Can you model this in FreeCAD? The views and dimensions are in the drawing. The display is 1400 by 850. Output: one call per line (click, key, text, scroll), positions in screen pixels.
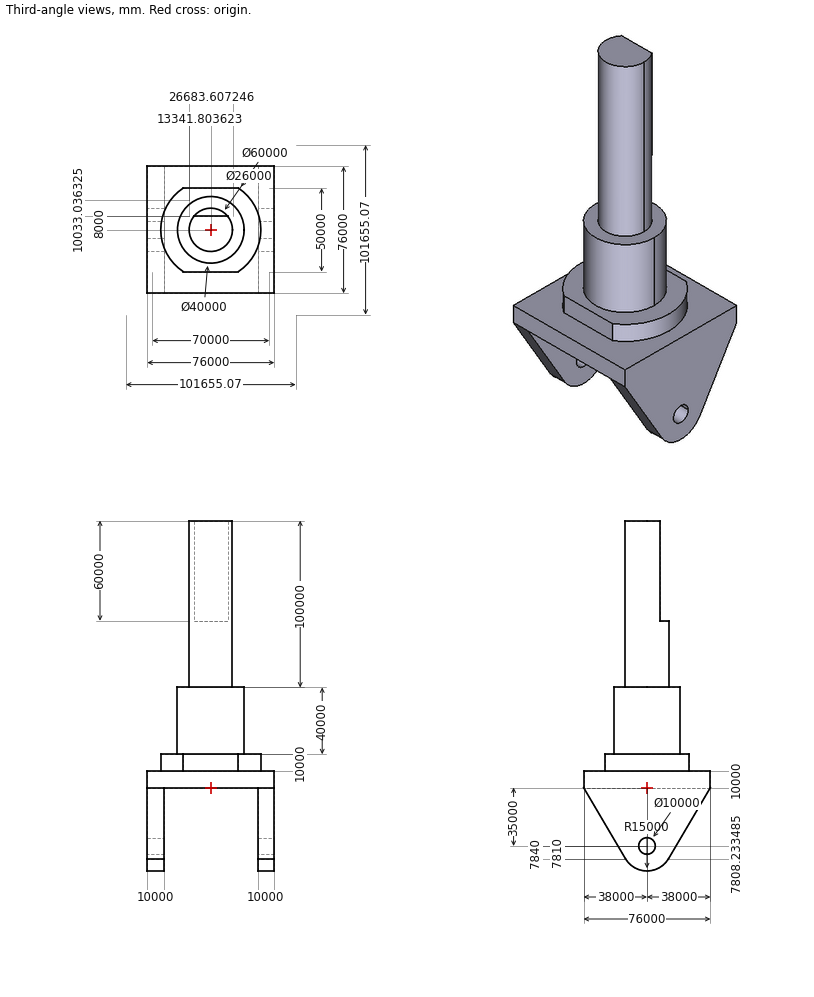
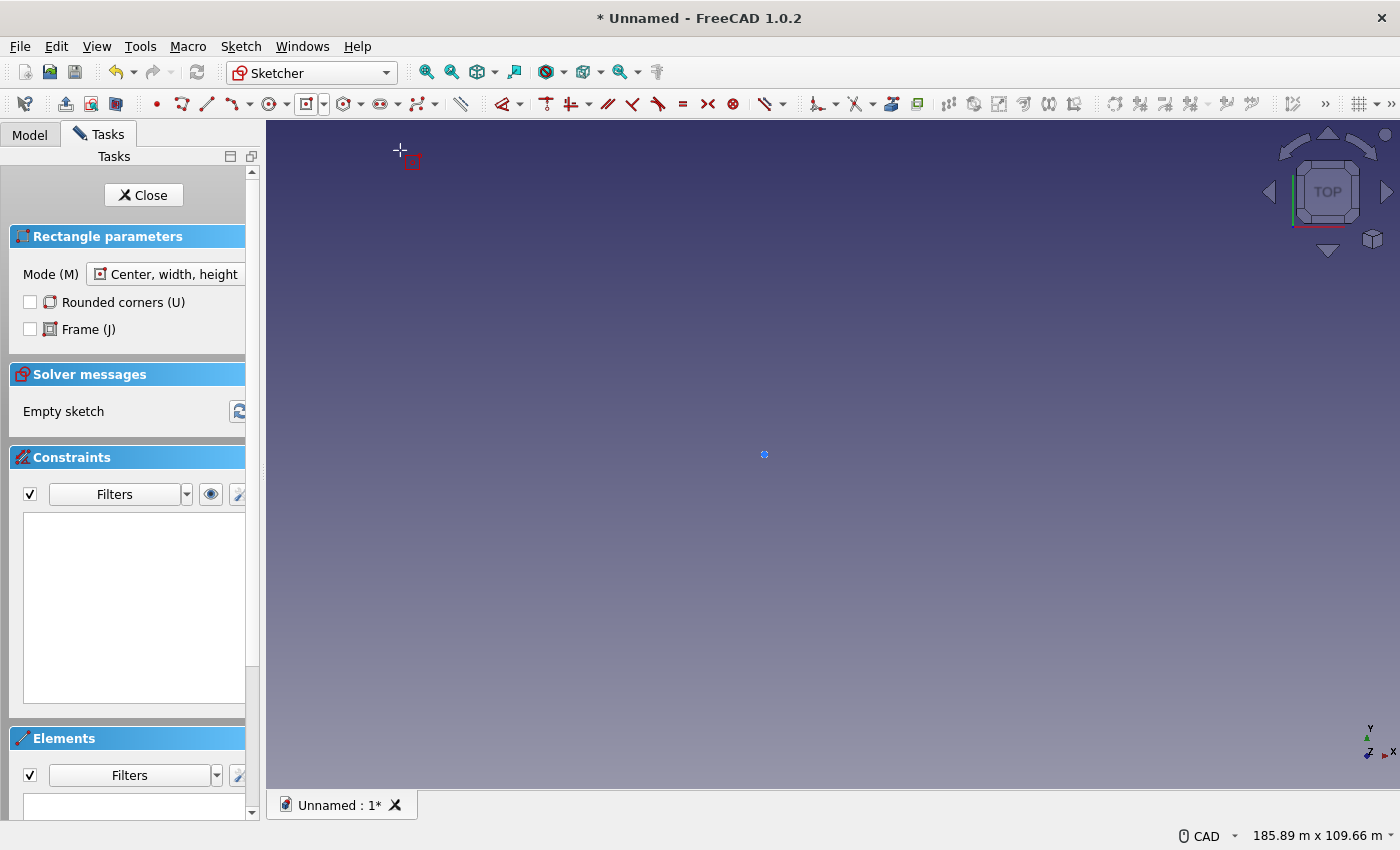
click(765, 454)
click(996, 223)
key(Escape)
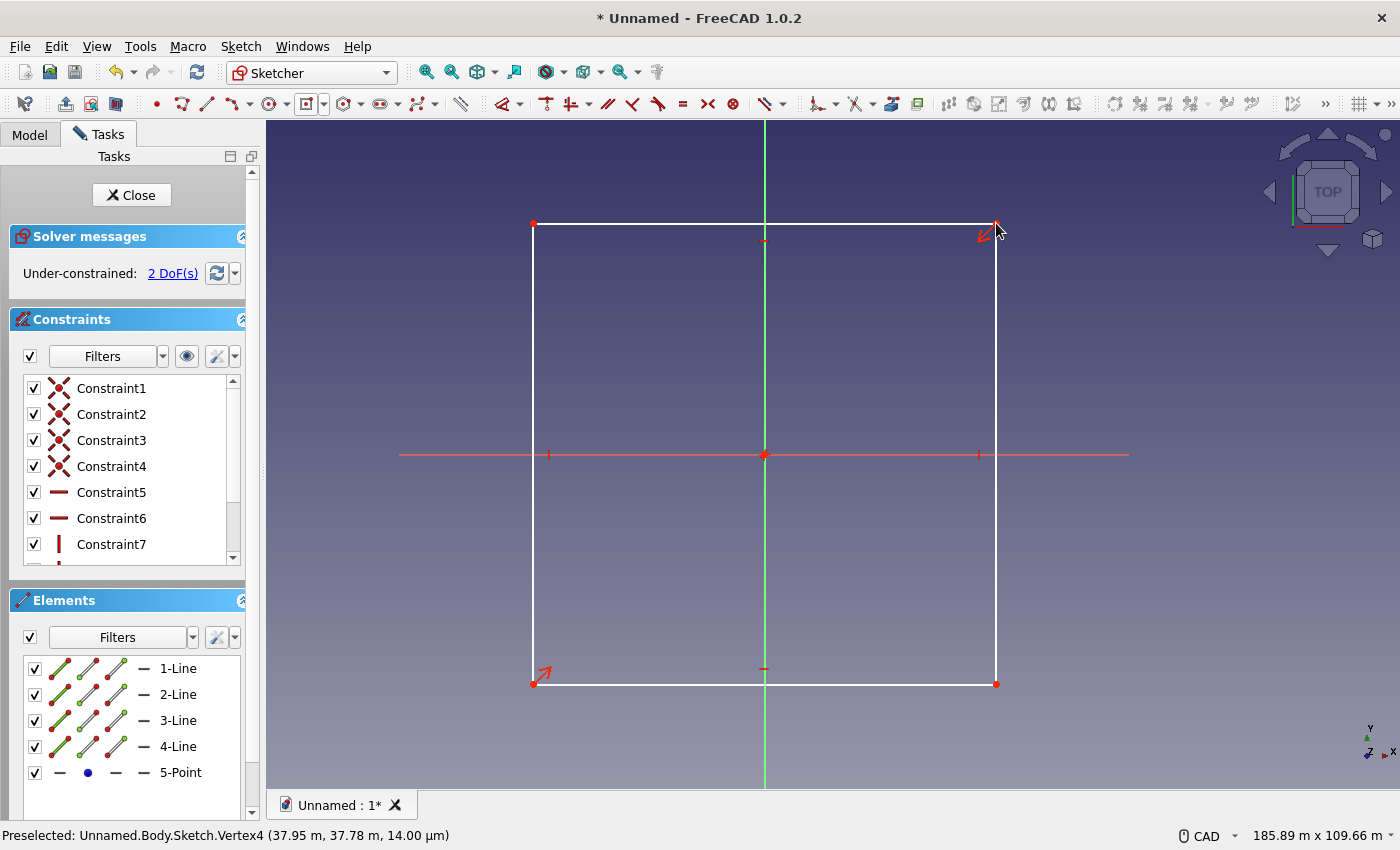
click(502, 104)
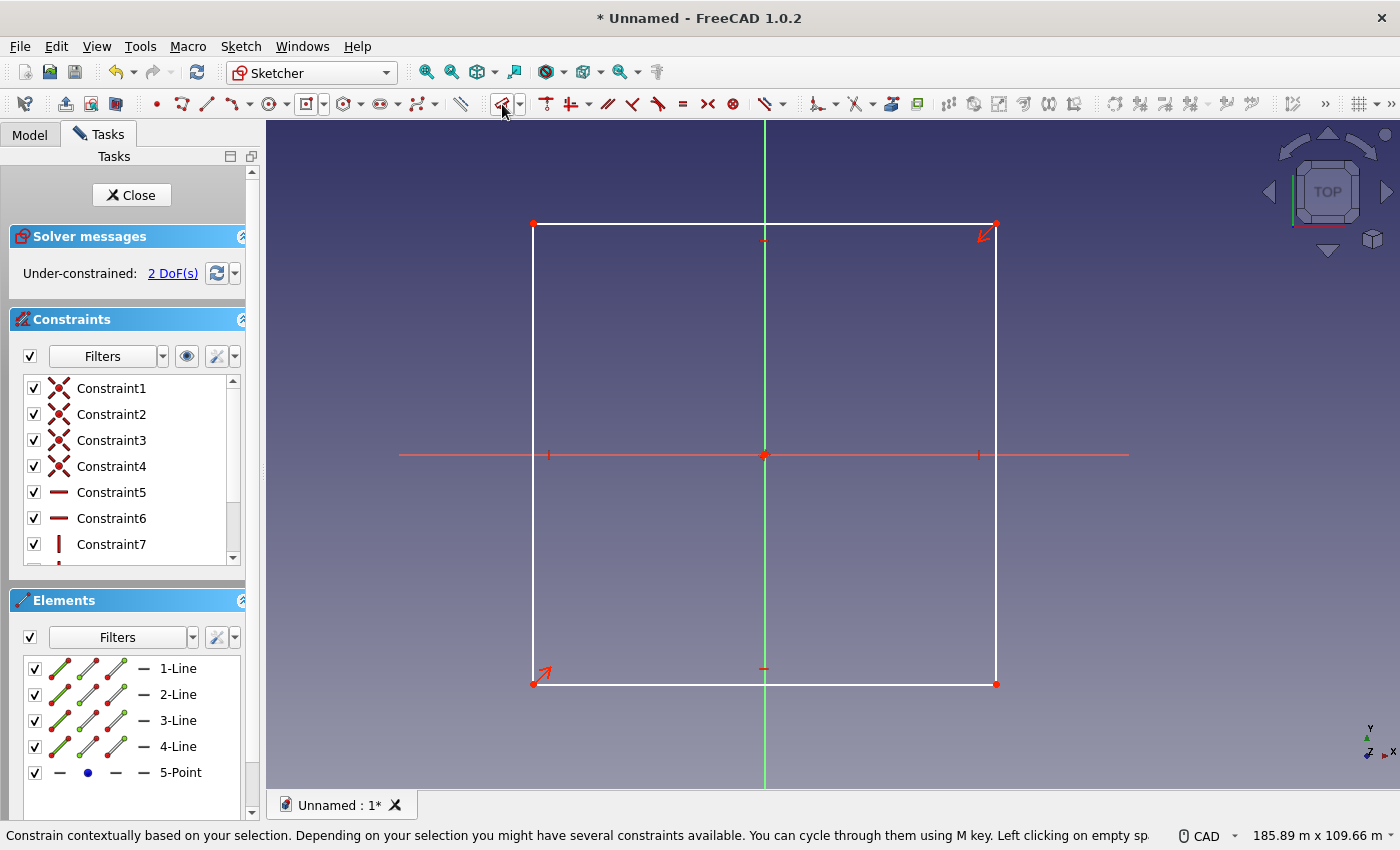
click(672, 685)
click(658, 719)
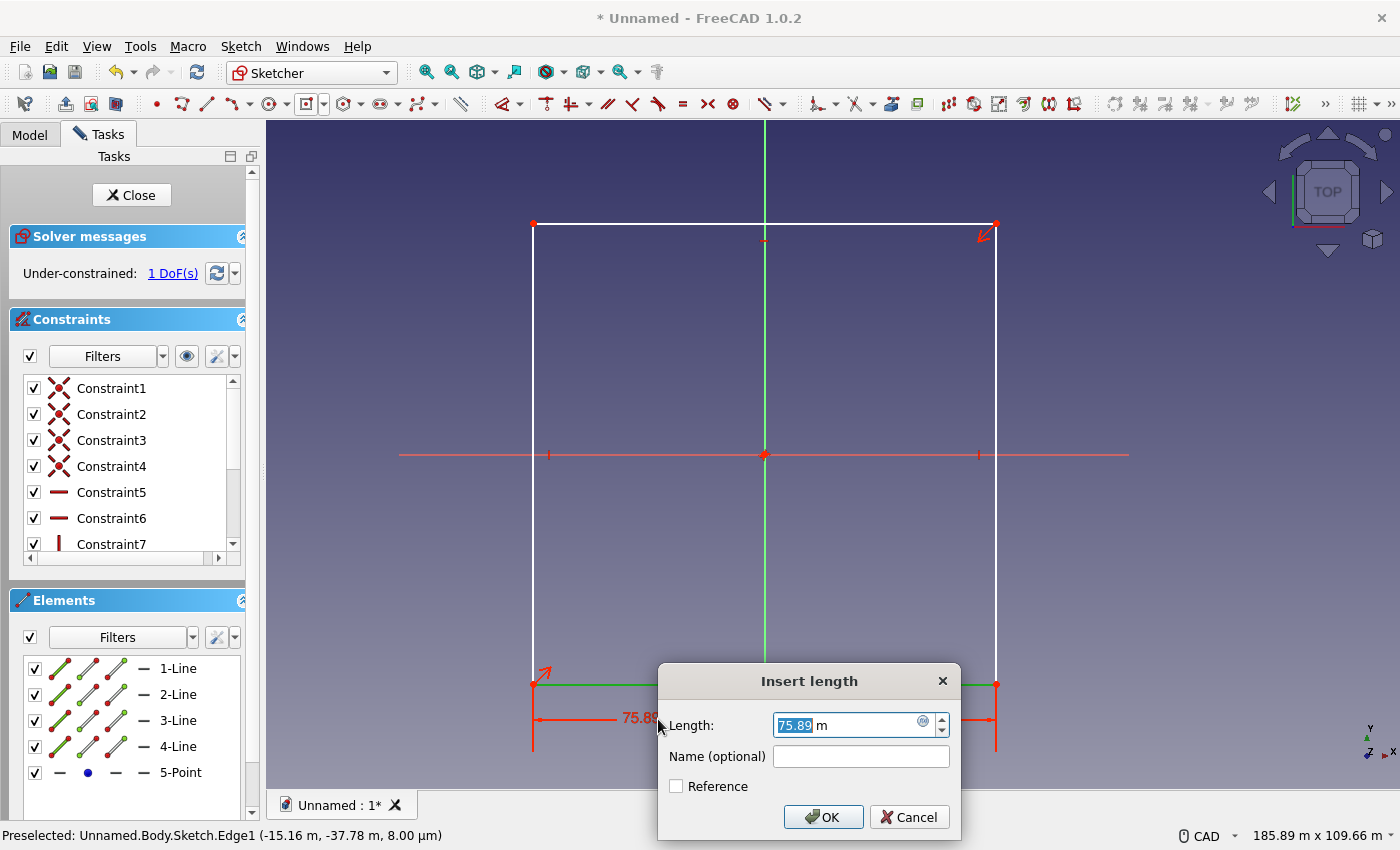
key(ctrl+a)
text(76000 mm)
key(Return)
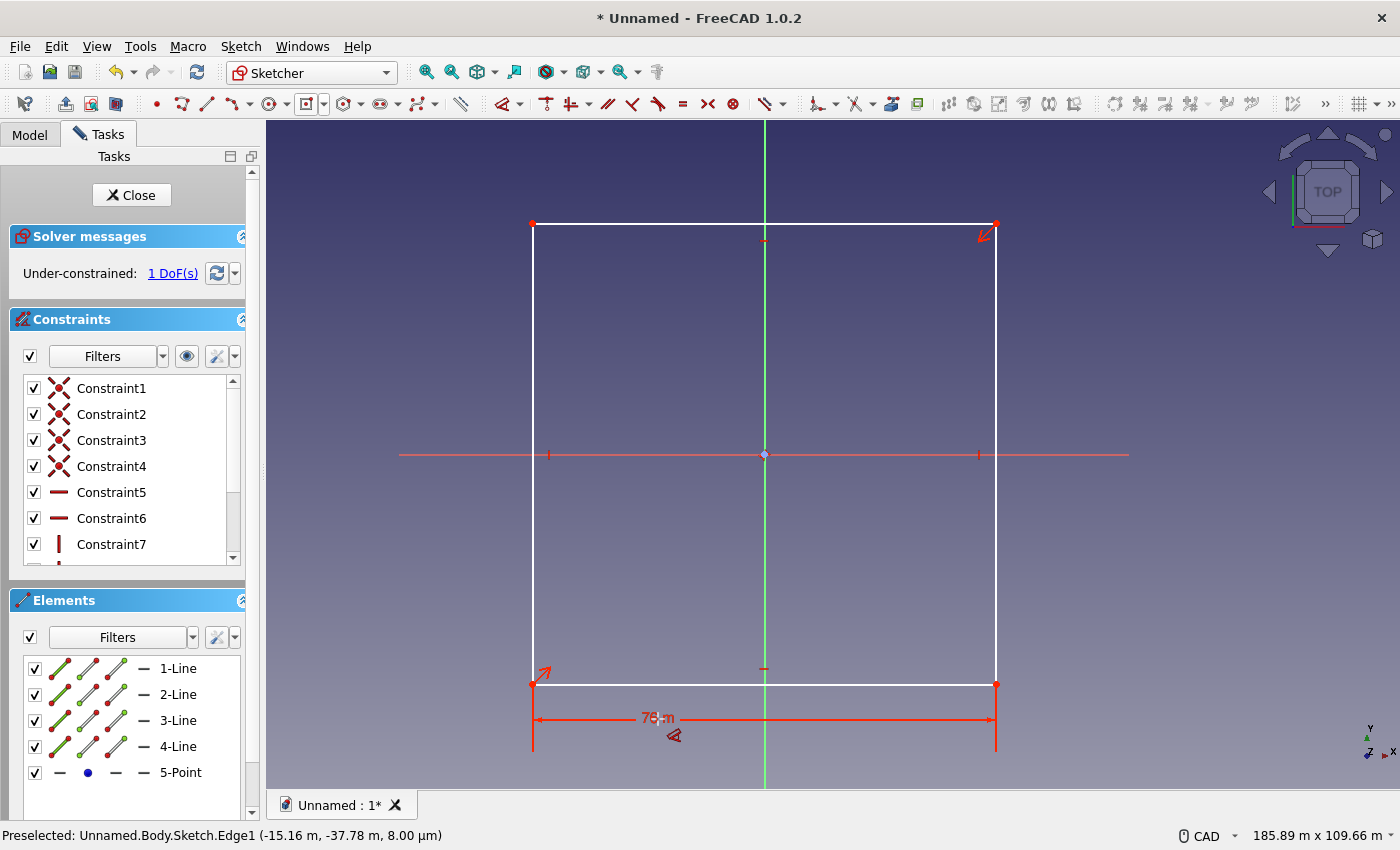
click(996, 547)
click(1030, 348)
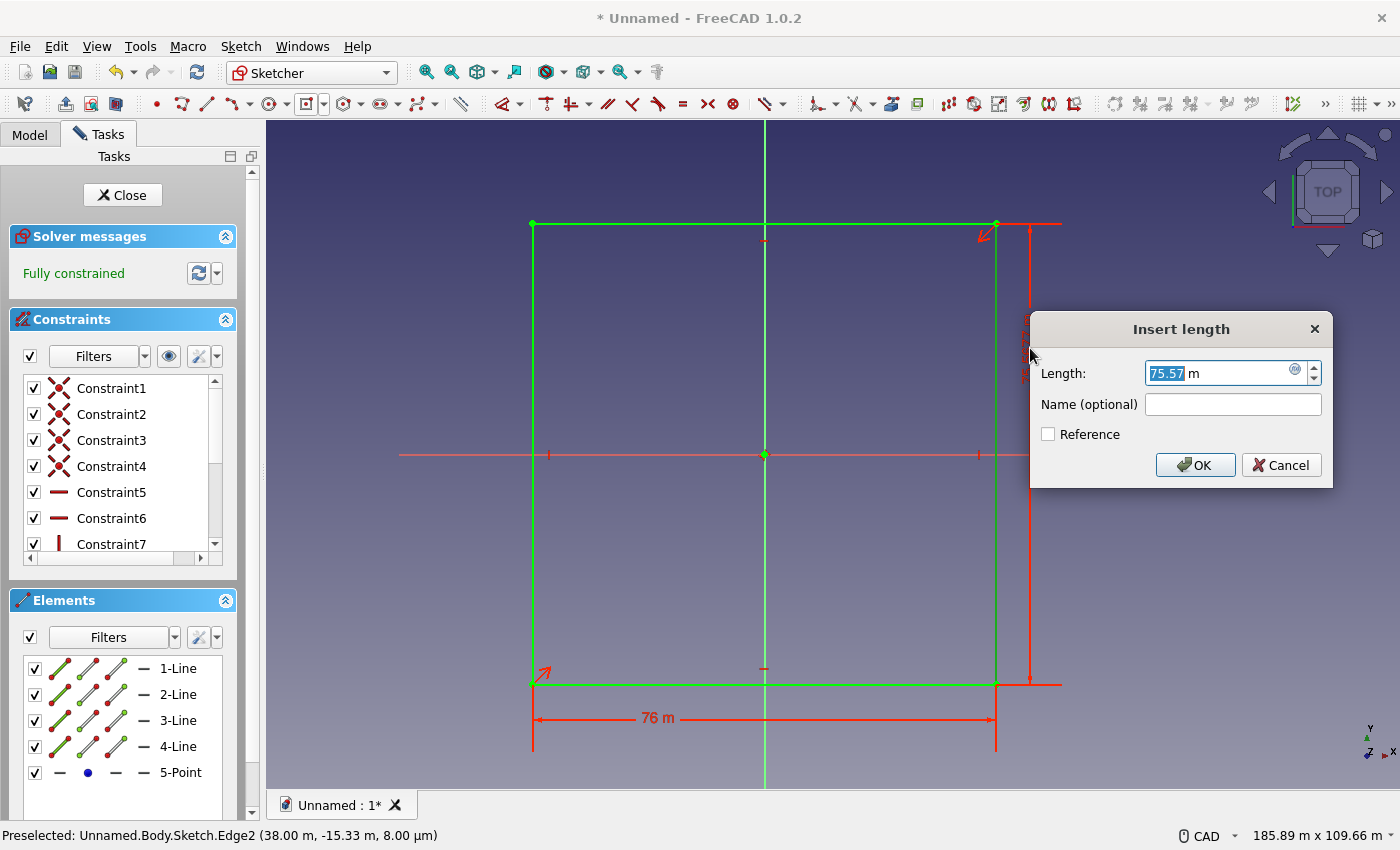
key(ctrl+a)
text(76000 mm)
key(Return)
key(Escape)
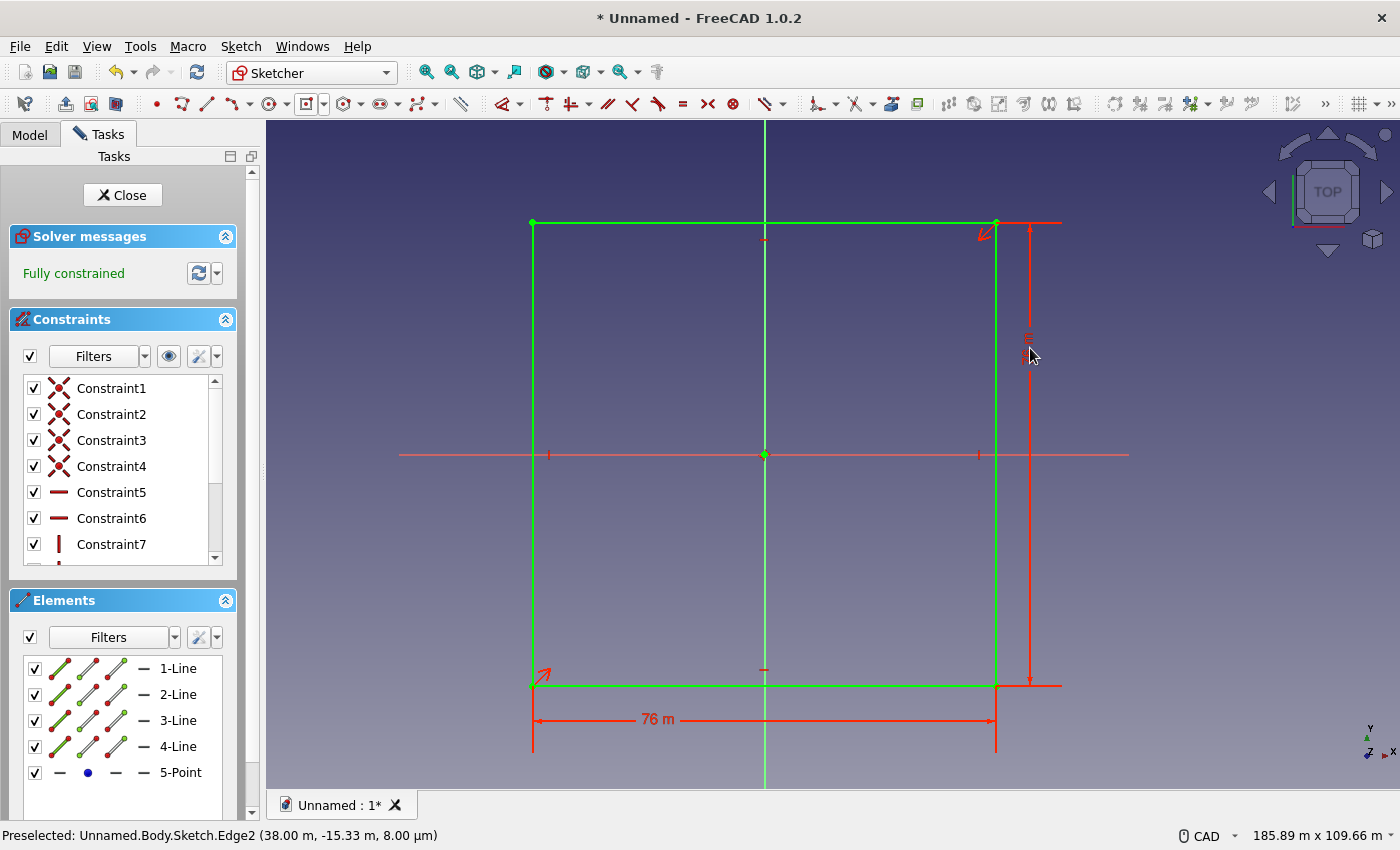
click(123, 195)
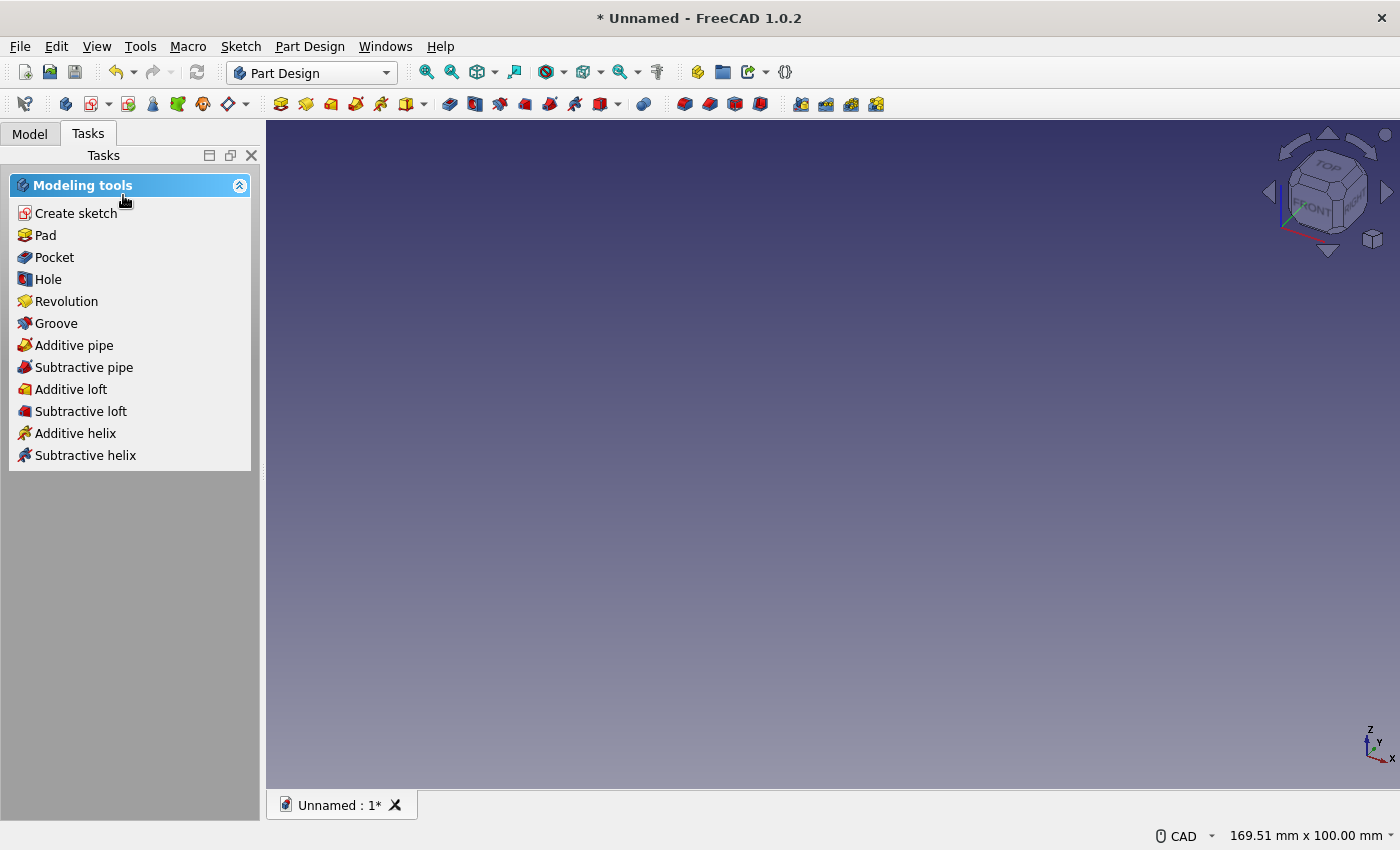
click(281, 104)